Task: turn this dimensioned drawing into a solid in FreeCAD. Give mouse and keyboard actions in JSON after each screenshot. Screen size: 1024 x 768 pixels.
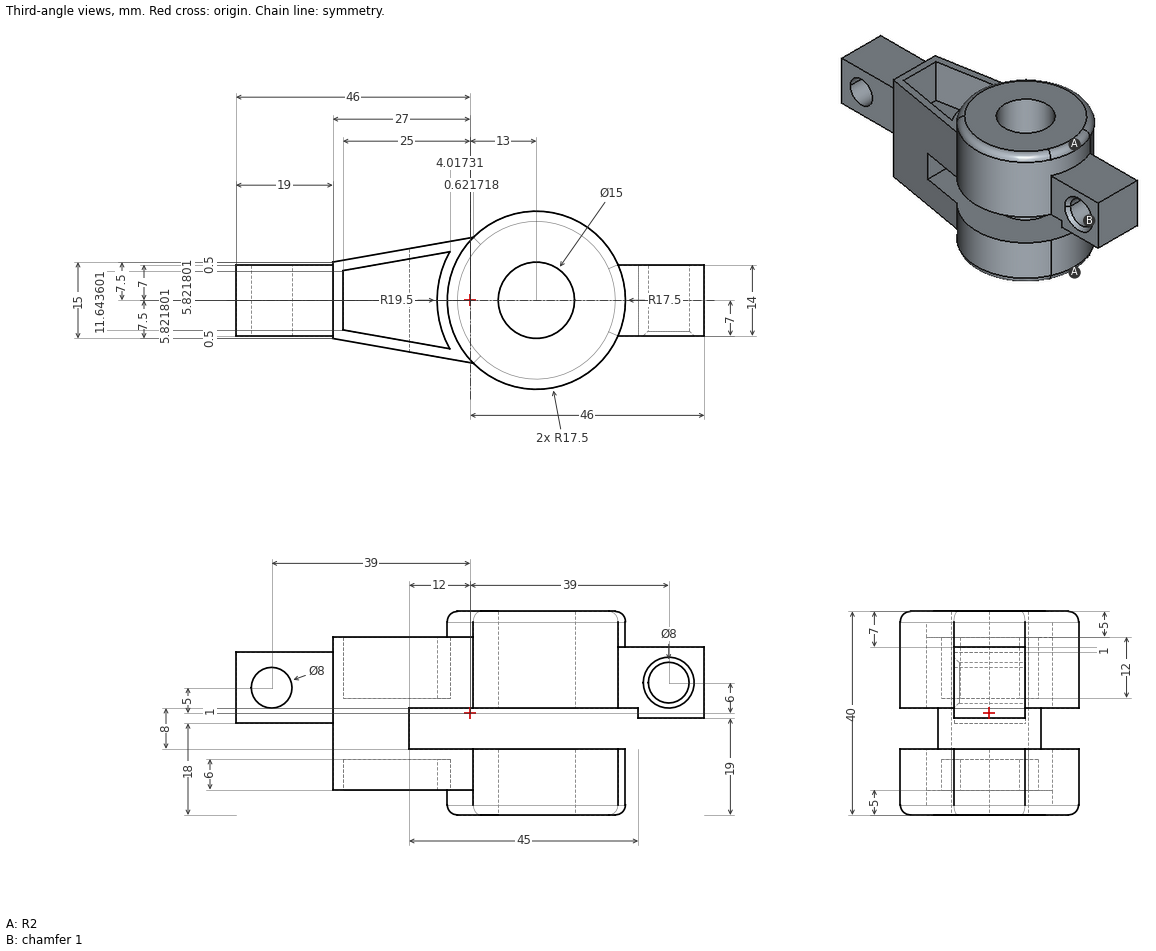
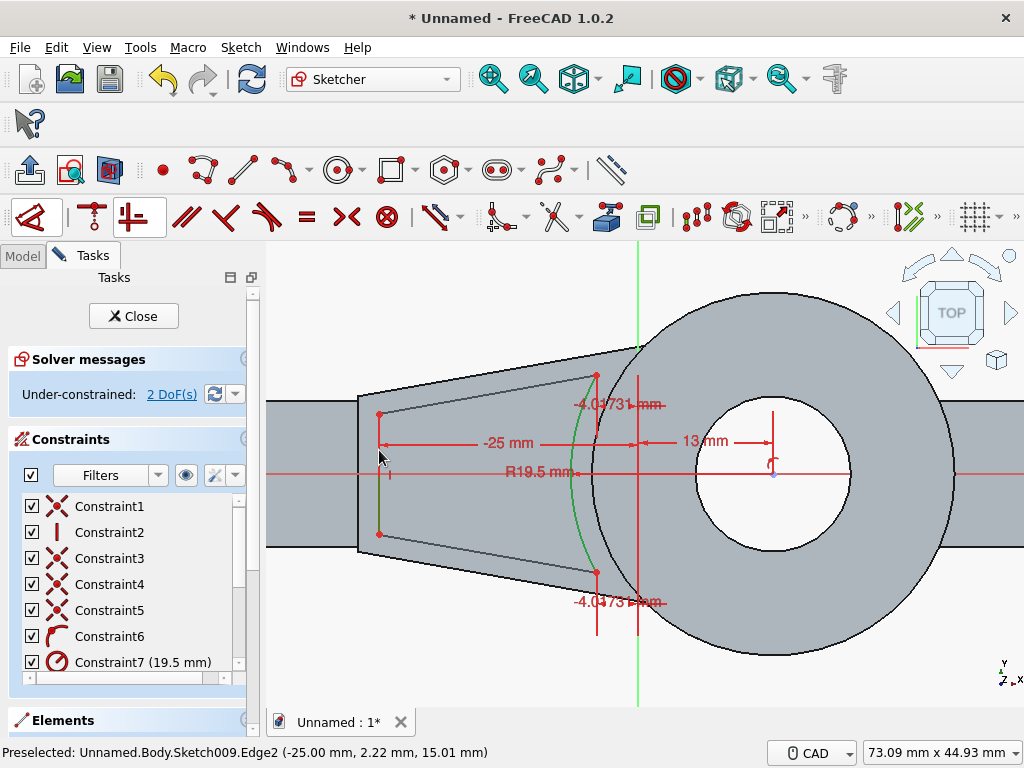
{"action": "key", "text": "i"}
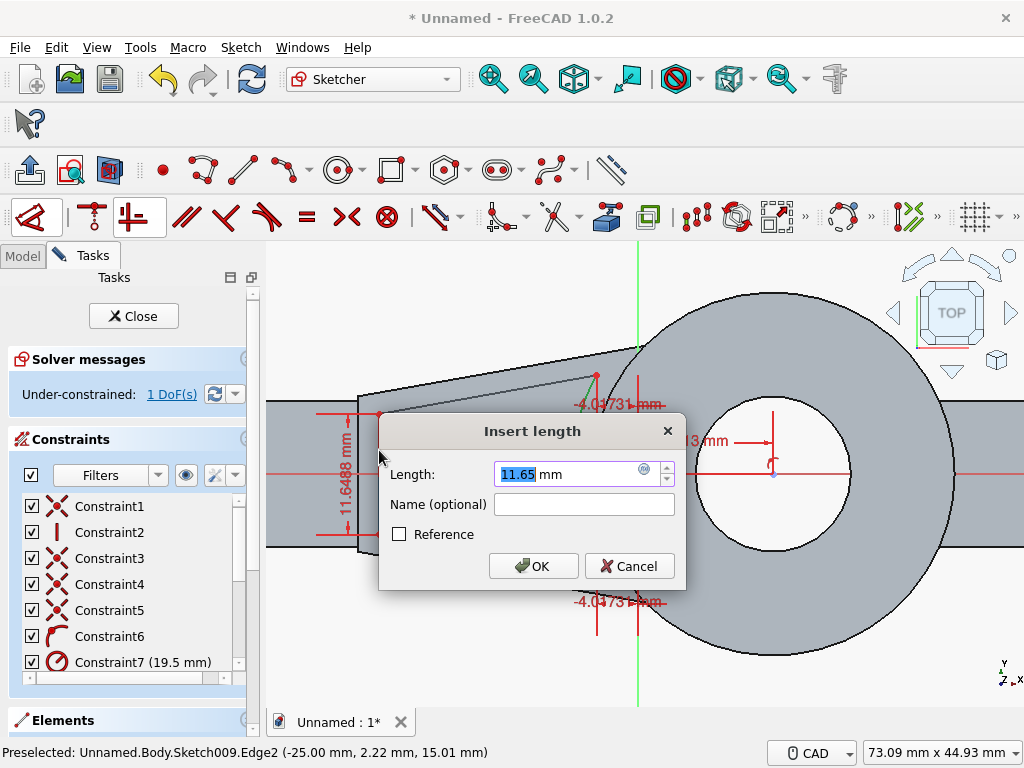
{"action": "type", "text": "11.643601"}
{"action": "key", "text": "Return"}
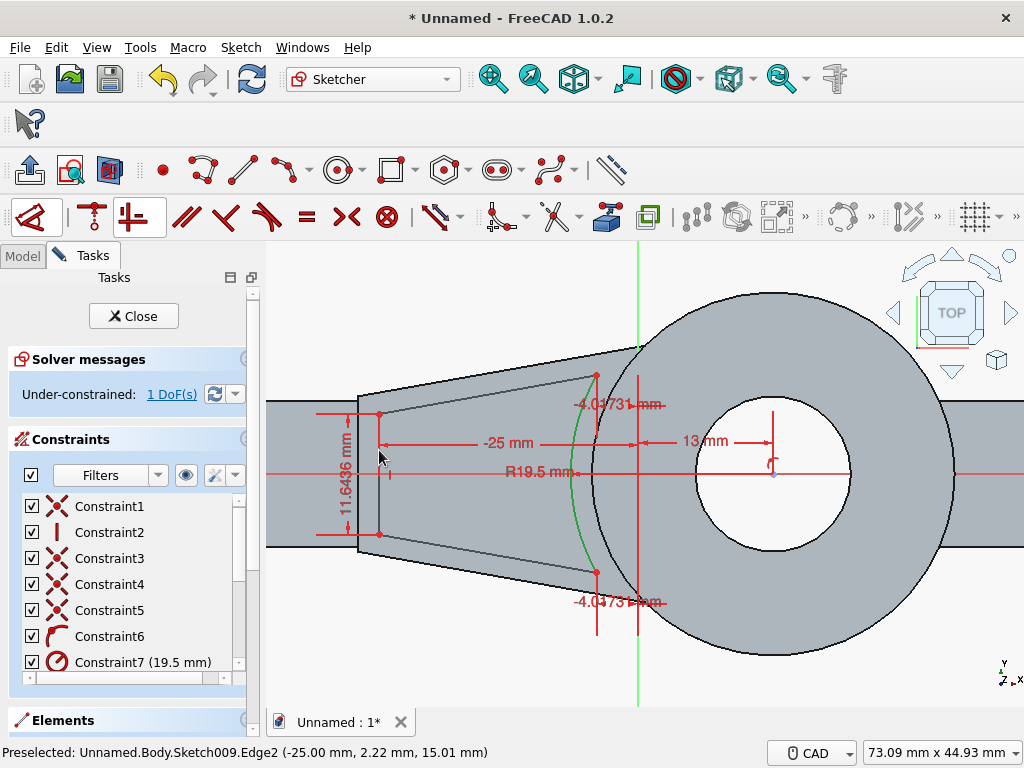
{"action": "left_click", "coordinate": [379, 414]}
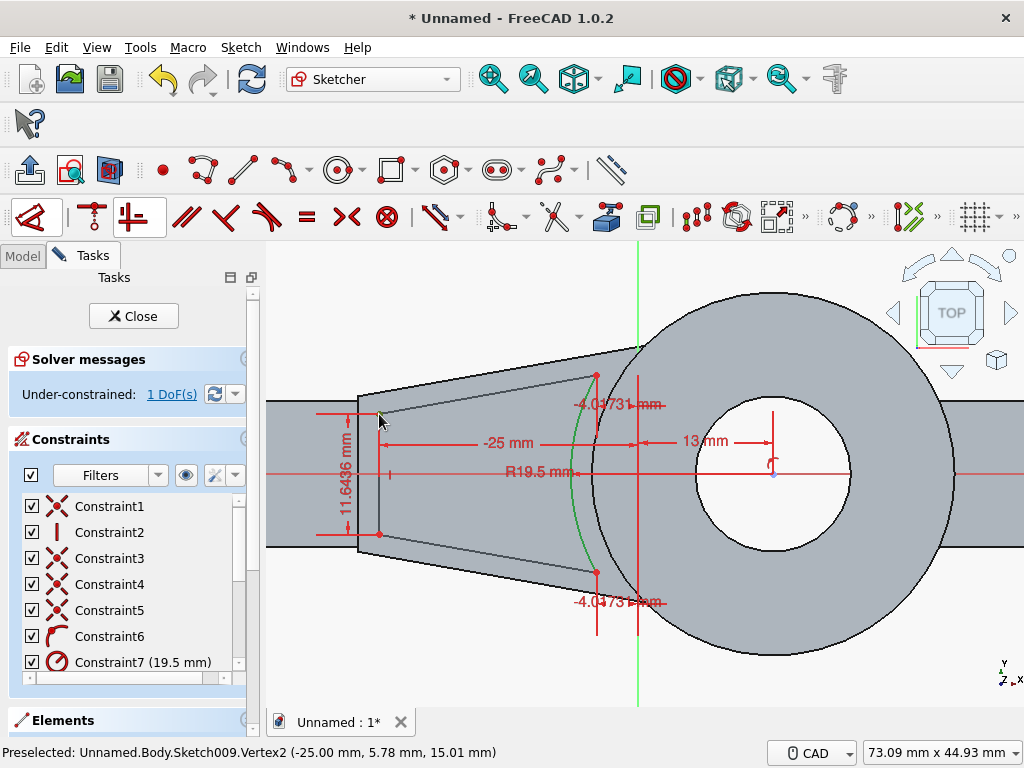
{"action": "key", "text": "i"}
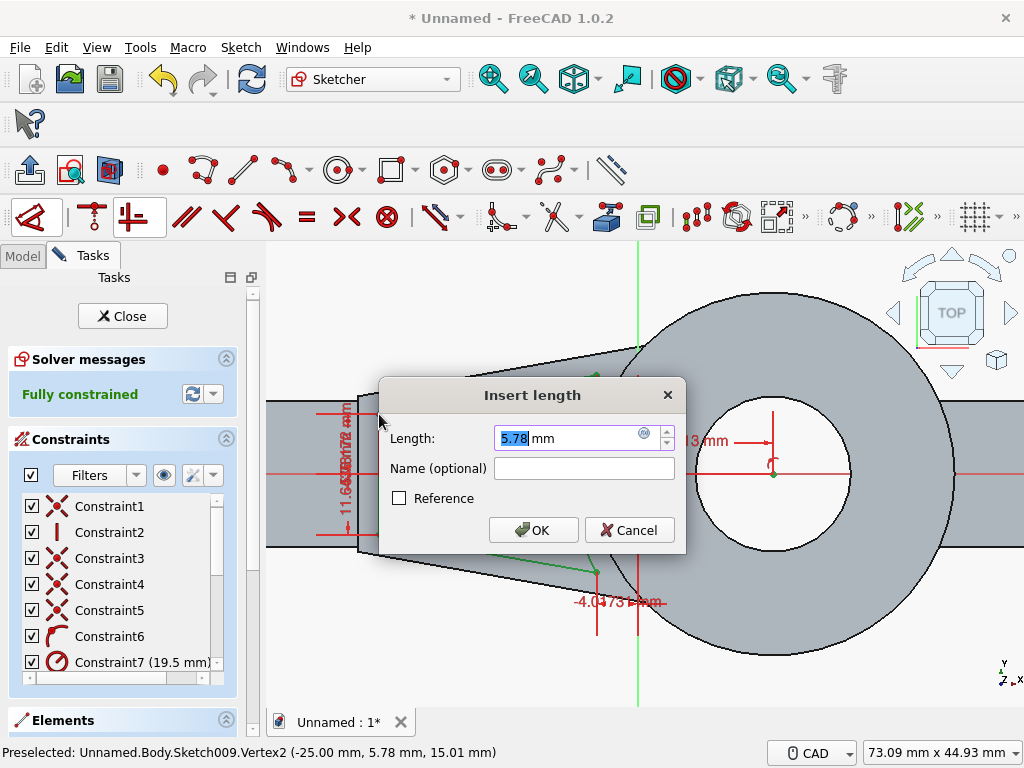
{"action": "type", "text": "5.821801"}
{"action": "key", "text": "Return"}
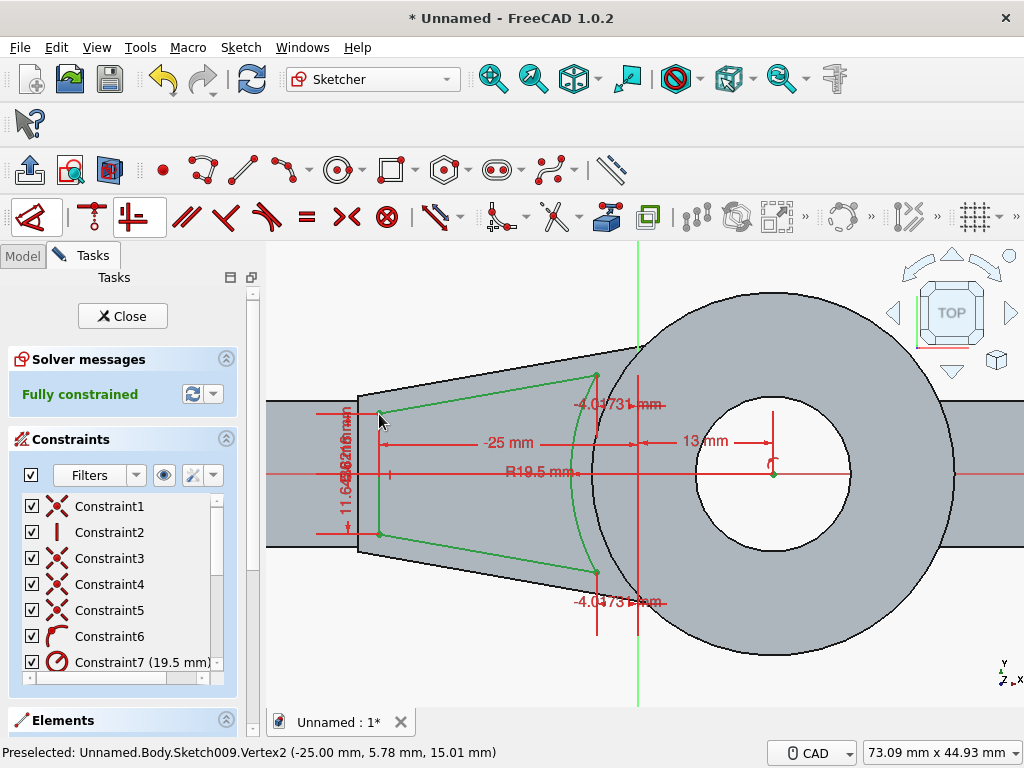
{"action": "left_click", "coordinate": [123, 316]}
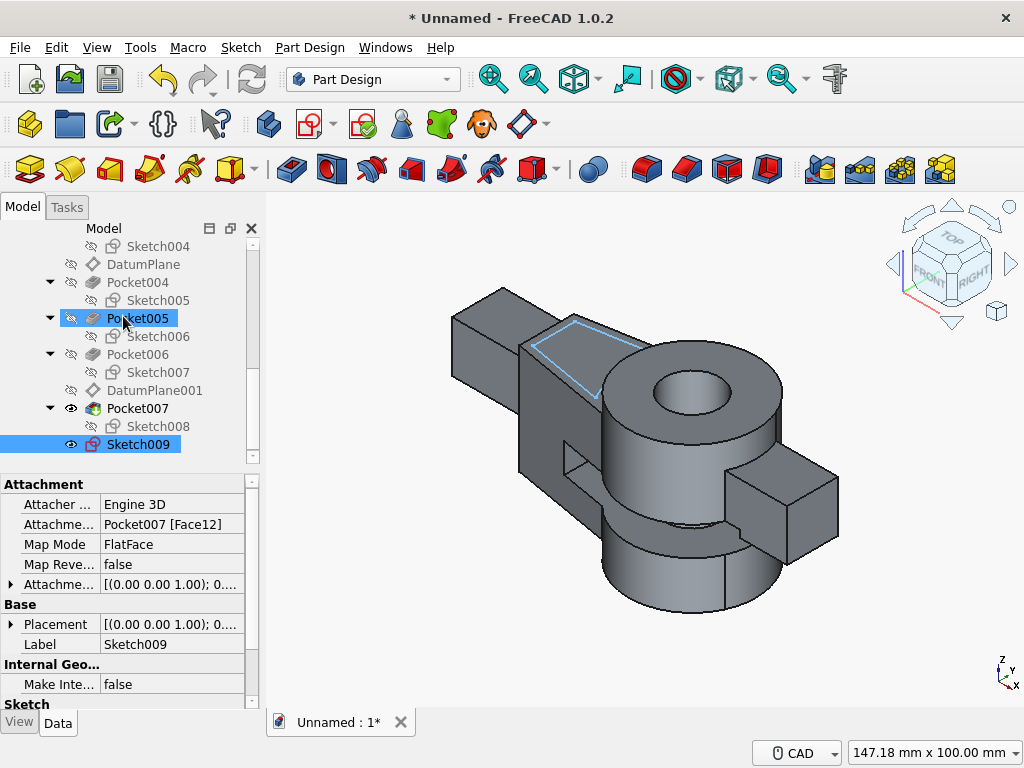
{"action": "left_click", "coordinate": [292, 170]}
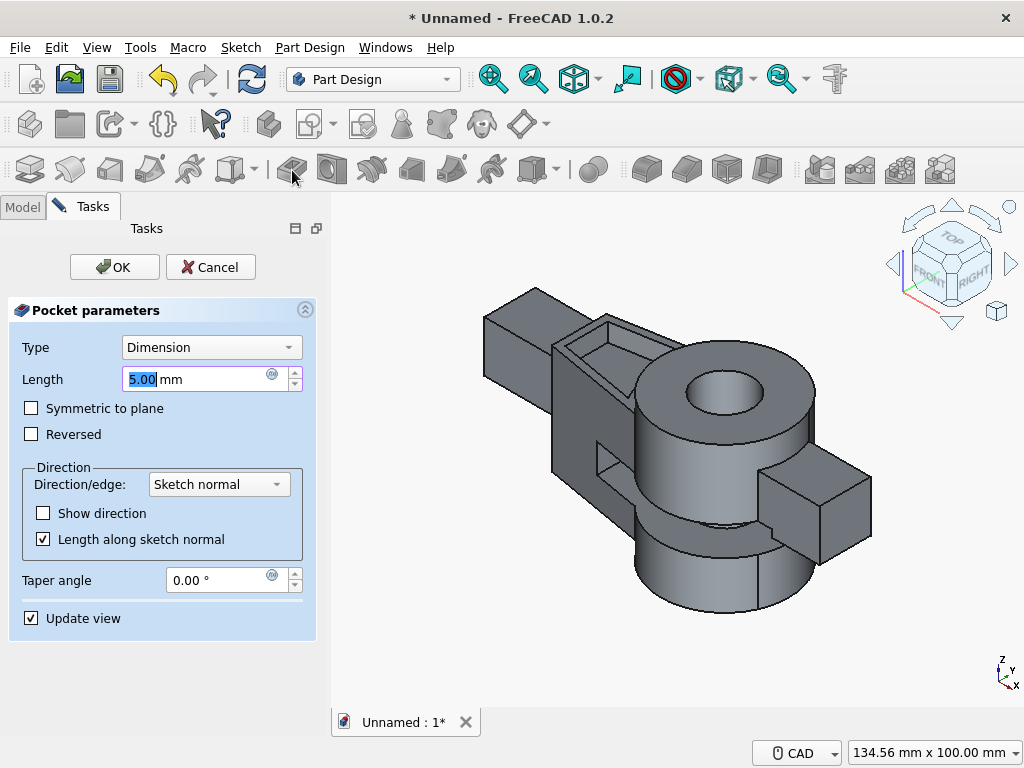
{"action": "type", "text": "12"}
{"action": "key", "text": "Tab"}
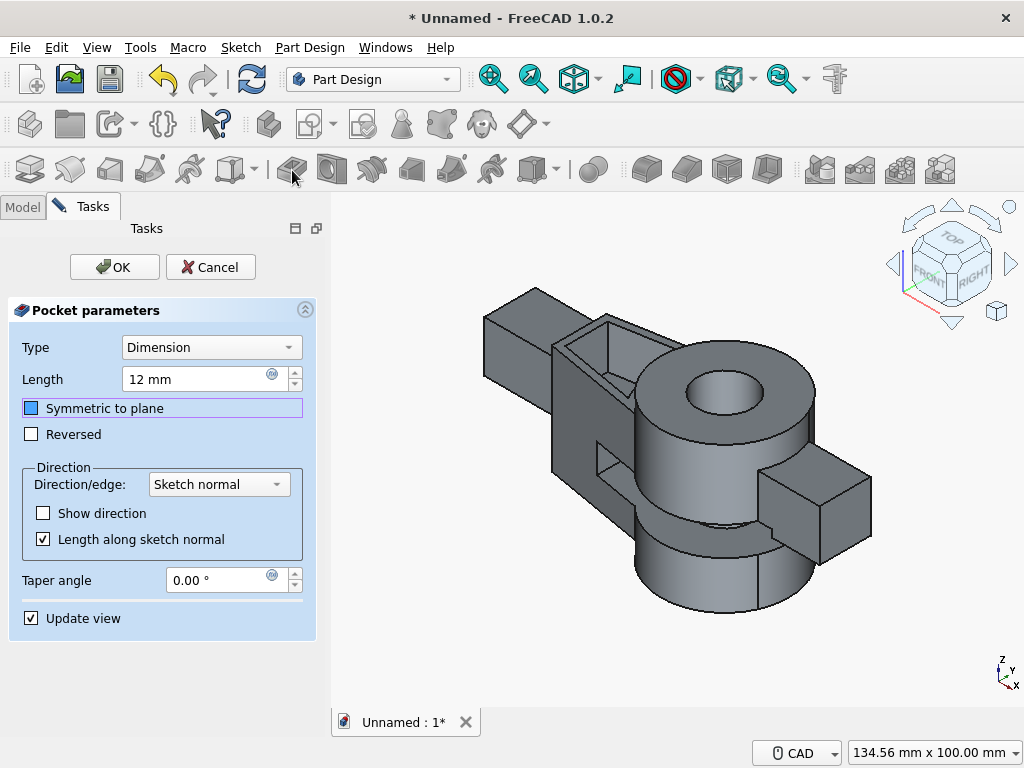
{"action": "left_click", "coordinate": [115, 267]}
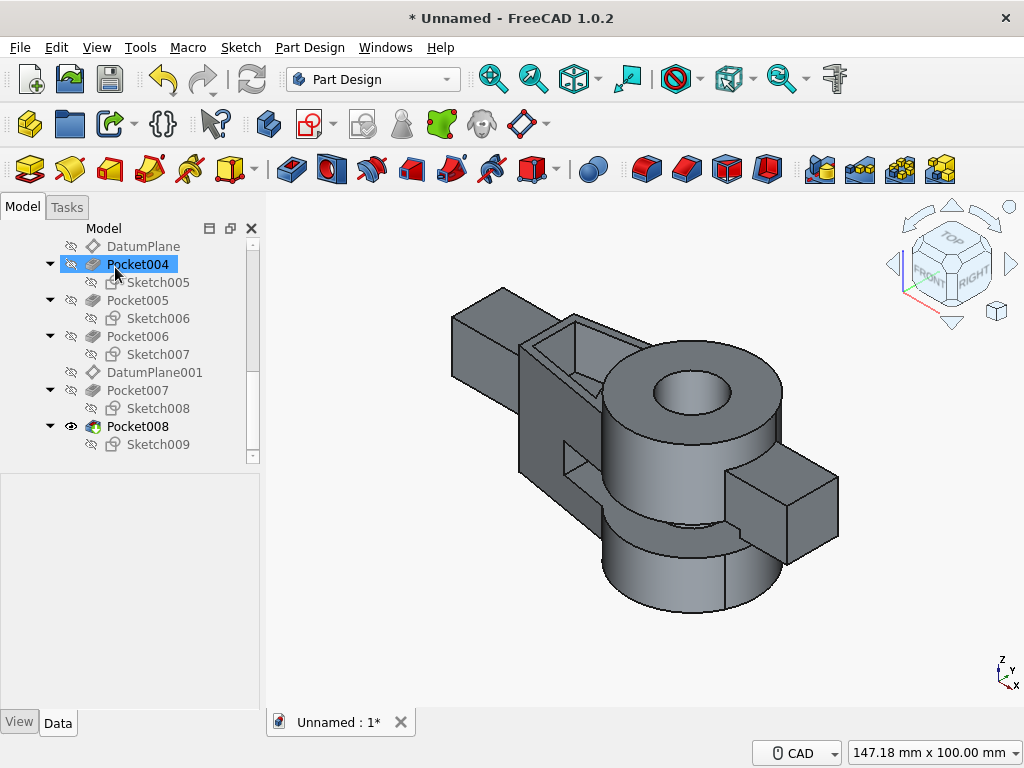
{"action": "scroll", "coordinate": [140, 350], "scroll_direction": "down", "scroll_amount": 3}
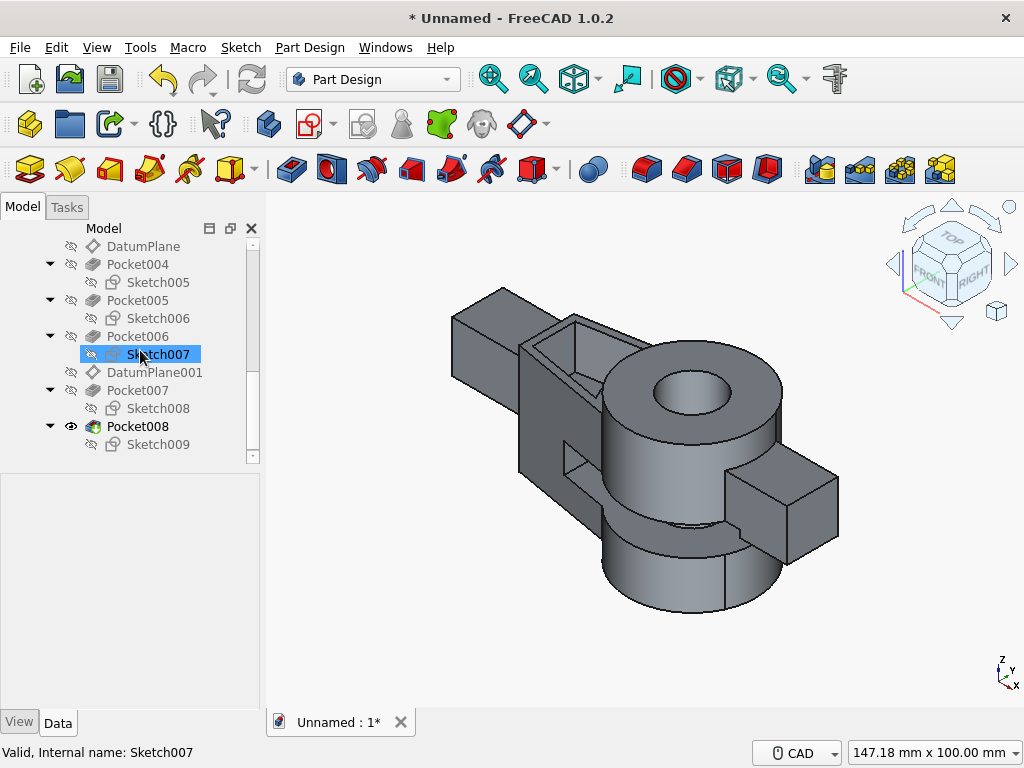
{"action": "scroll", "coordinate": [140, 350], "scroll_direction": "up", "scroll_amount": 15}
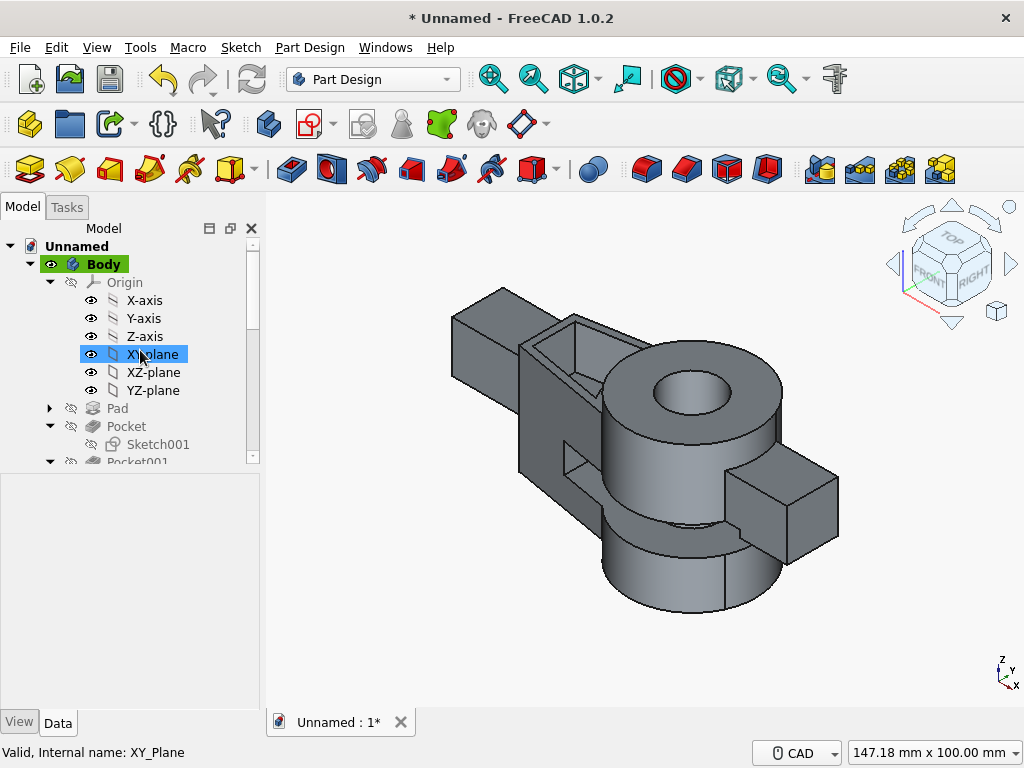
{"action": "left_click", "coordinate": [136, 354]}